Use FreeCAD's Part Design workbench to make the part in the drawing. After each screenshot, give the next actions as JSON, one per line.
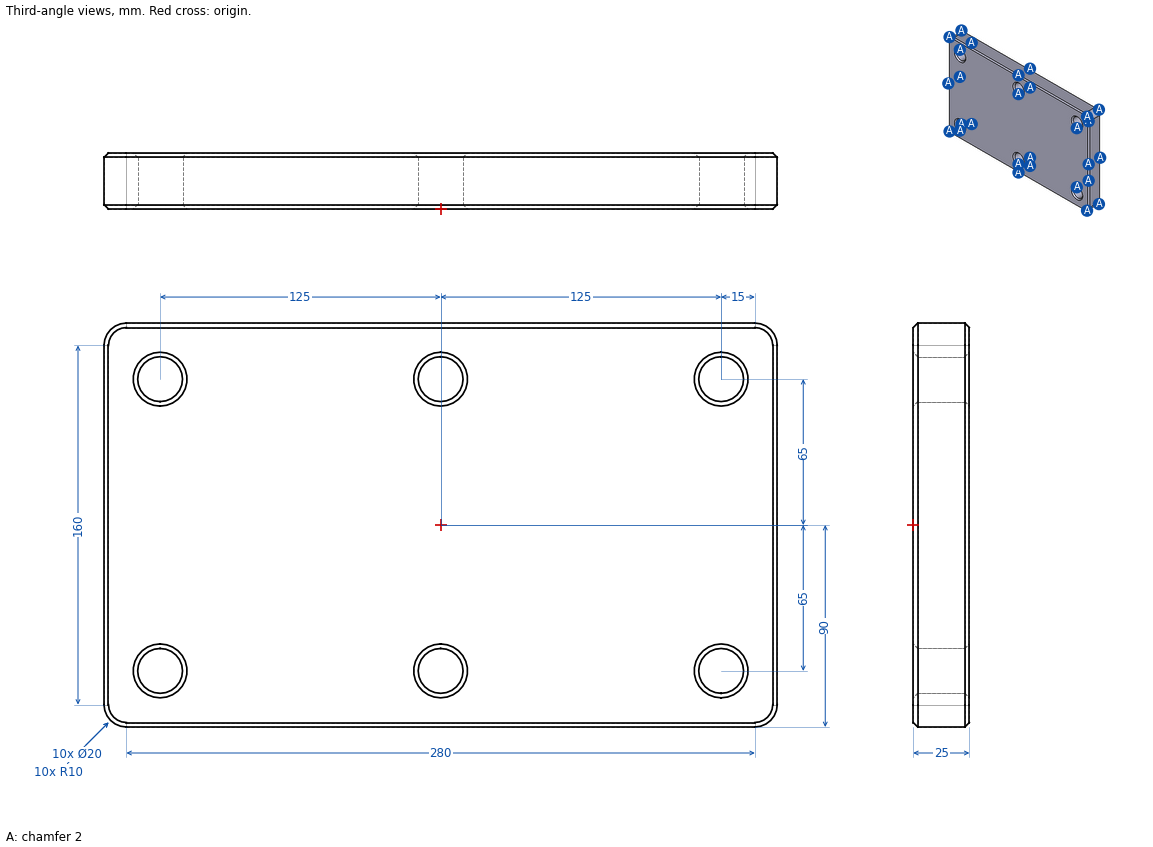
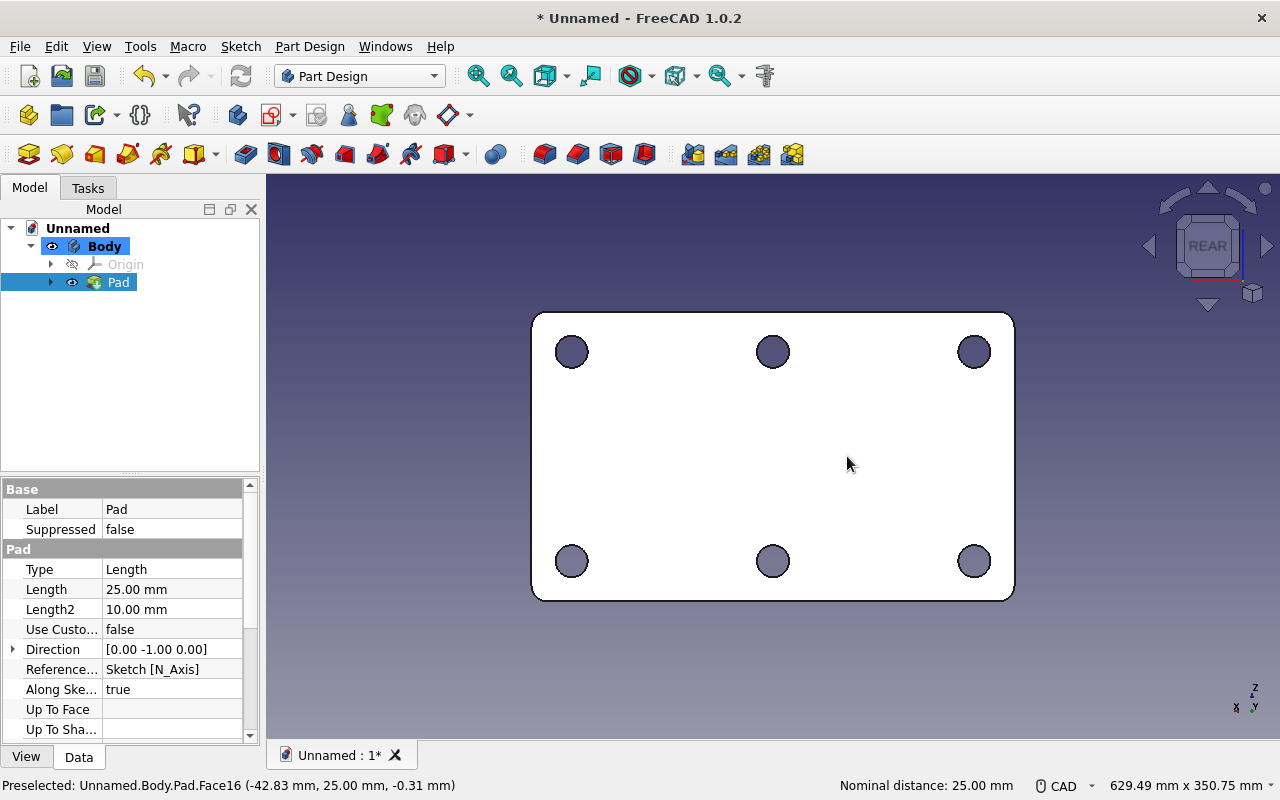
{"action": "left_click", "coordinate": [578, 154]}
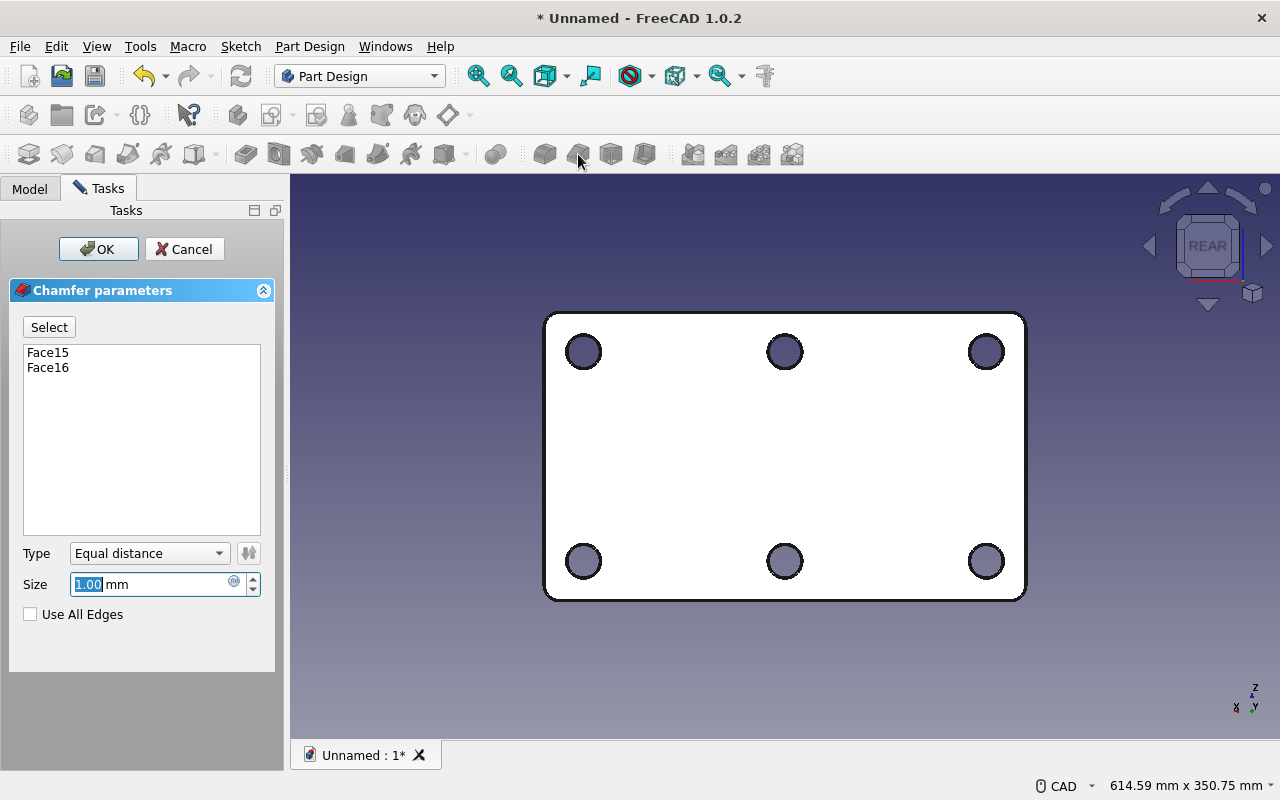
{"action": "type", "text": "2"}
{"action": "key", "text": "Tab"}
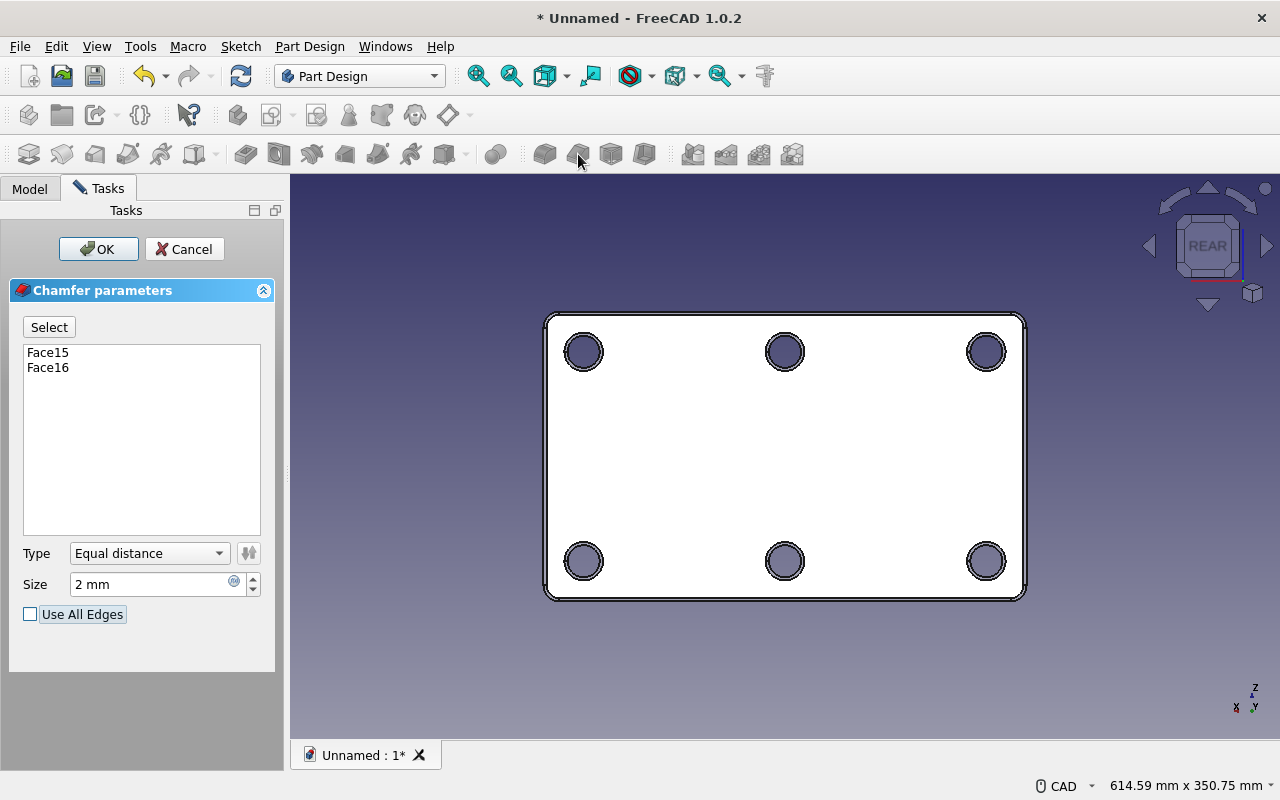
{"action": "left_click", "coordinate": [99, 249]}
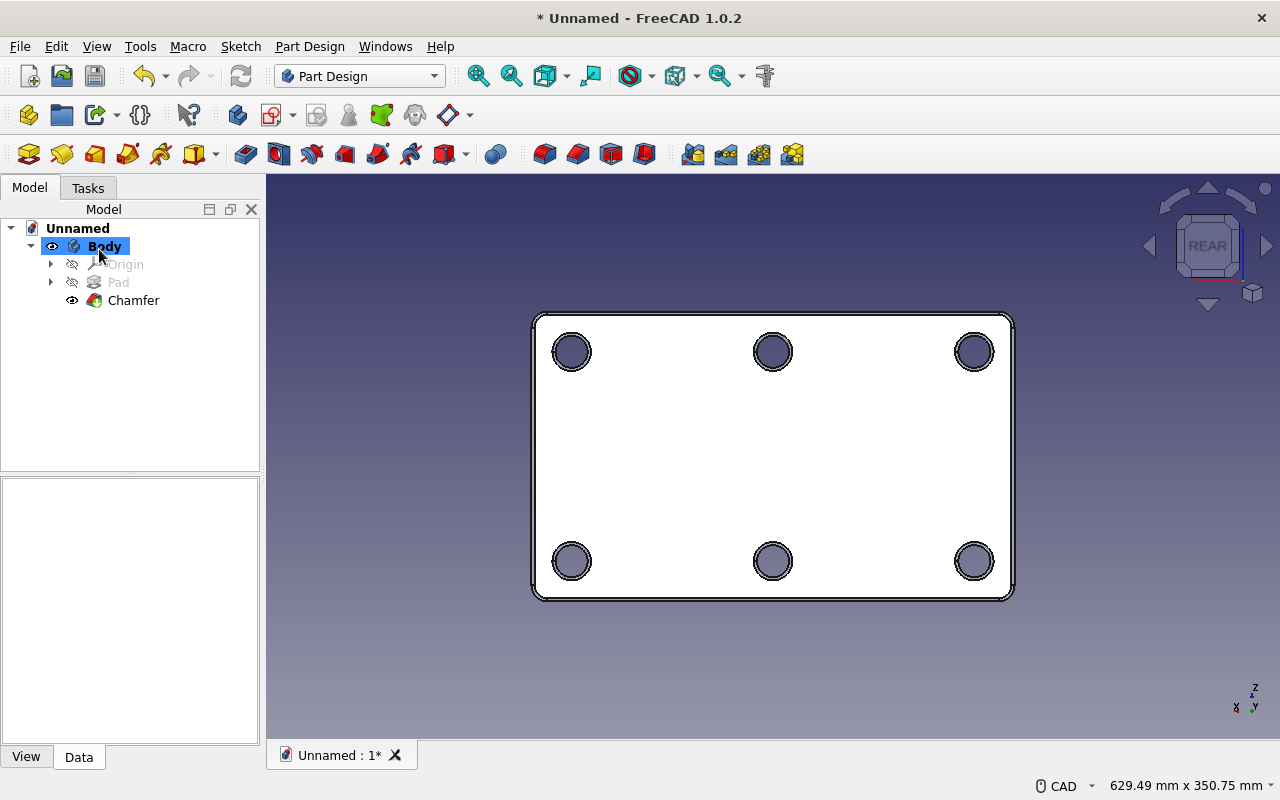
{"action": "key", "text": "0"}